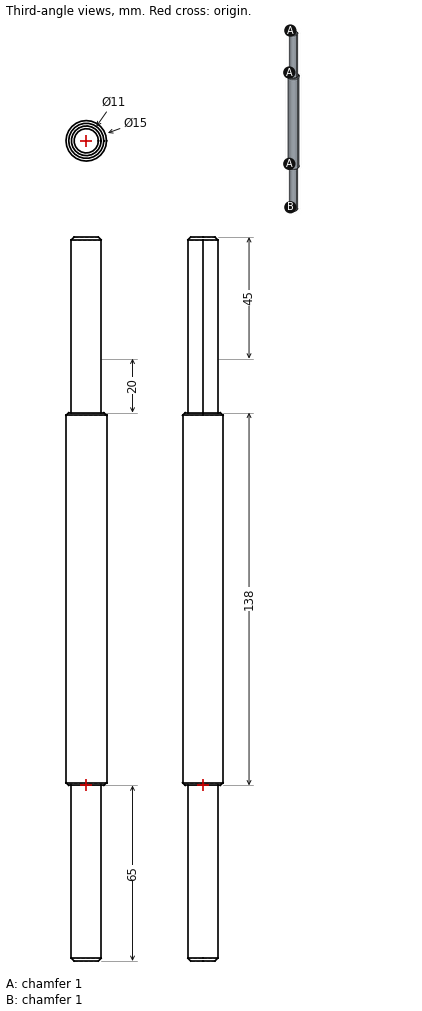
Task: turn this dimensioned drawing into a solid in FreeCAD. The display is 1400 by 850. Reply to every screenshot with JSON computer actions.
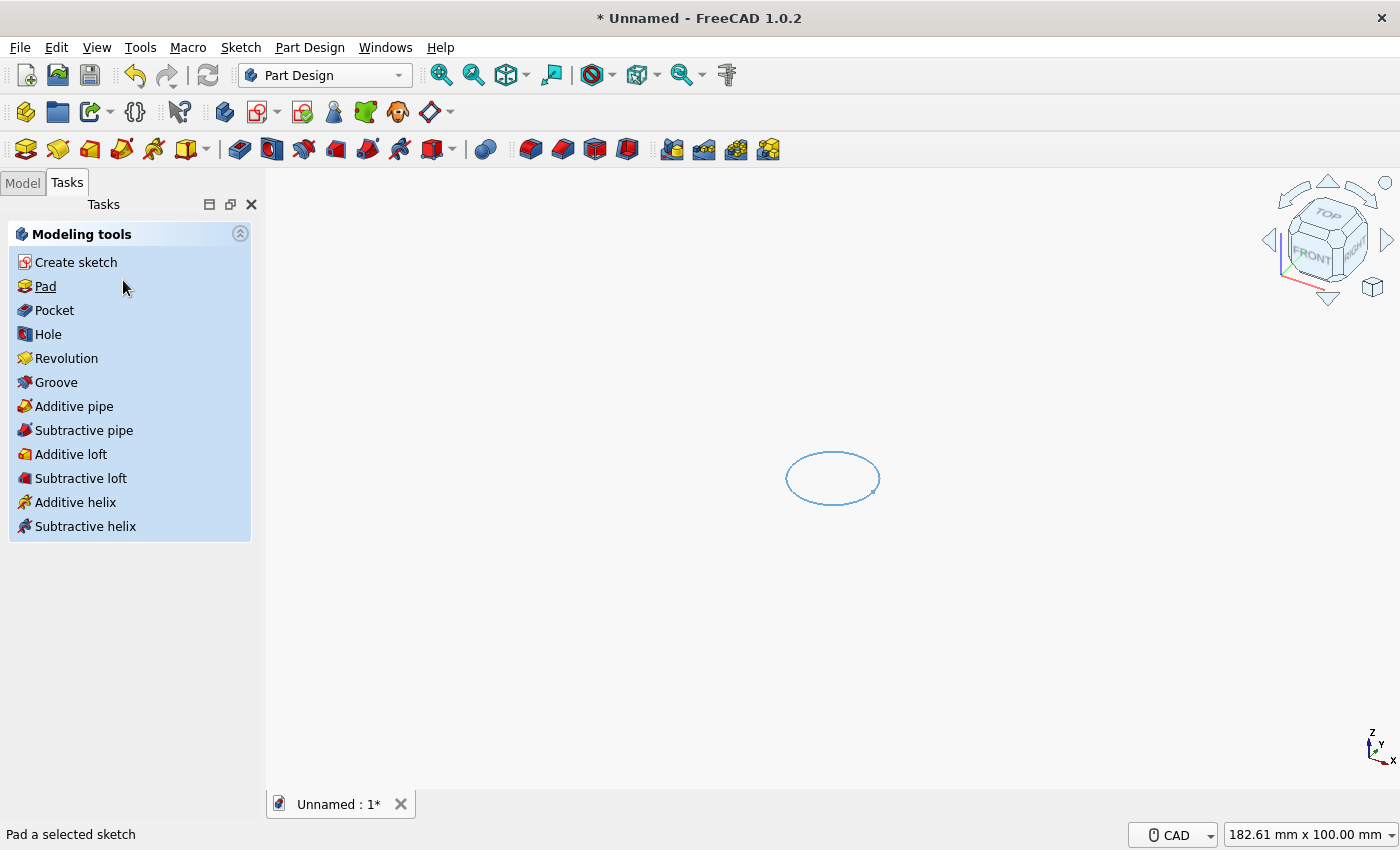
{"action": "left_click", "coordinate": [26, 150]}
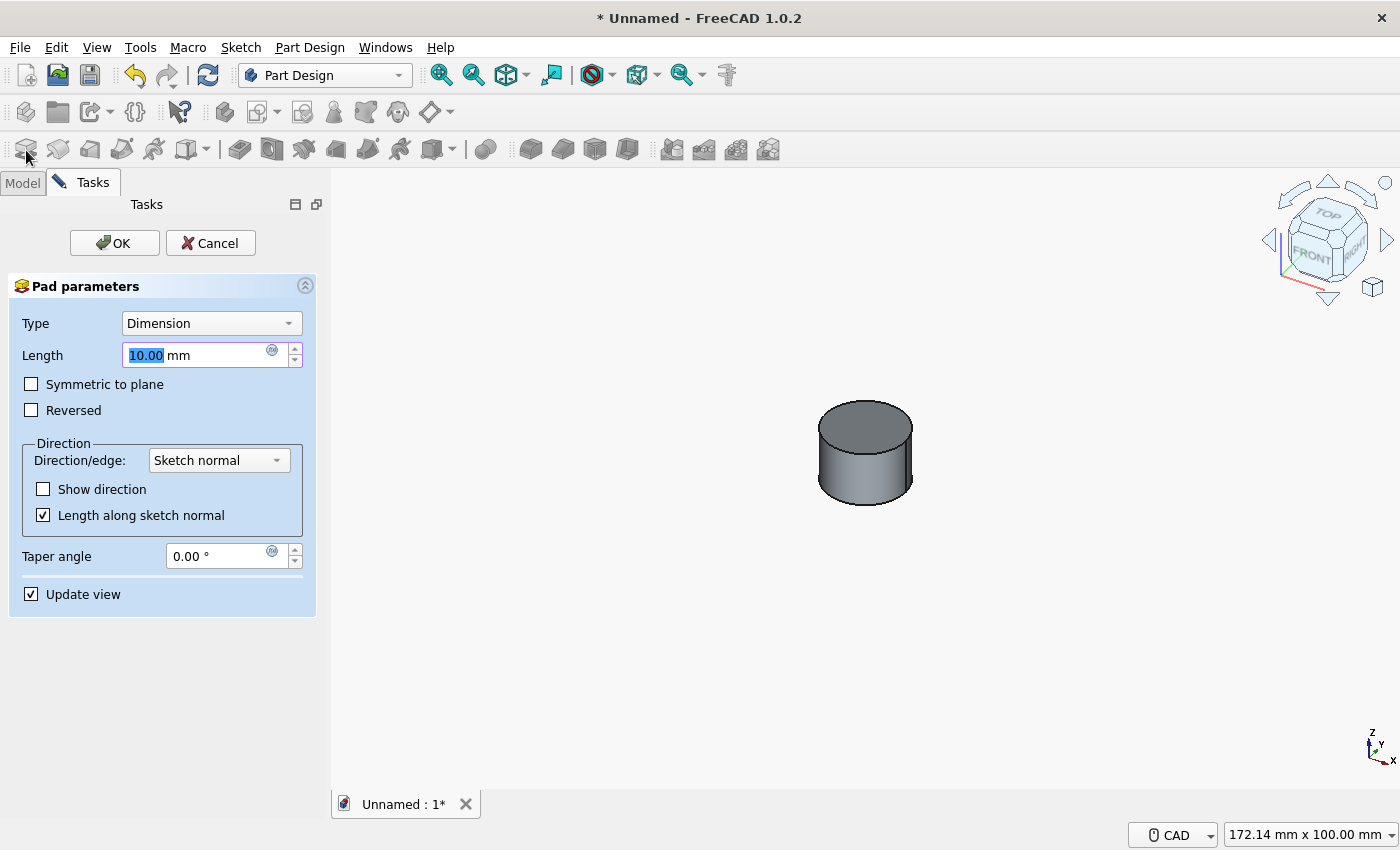
{"action": "type", "text": "138"}
{"action": "key", "text": "Tab"}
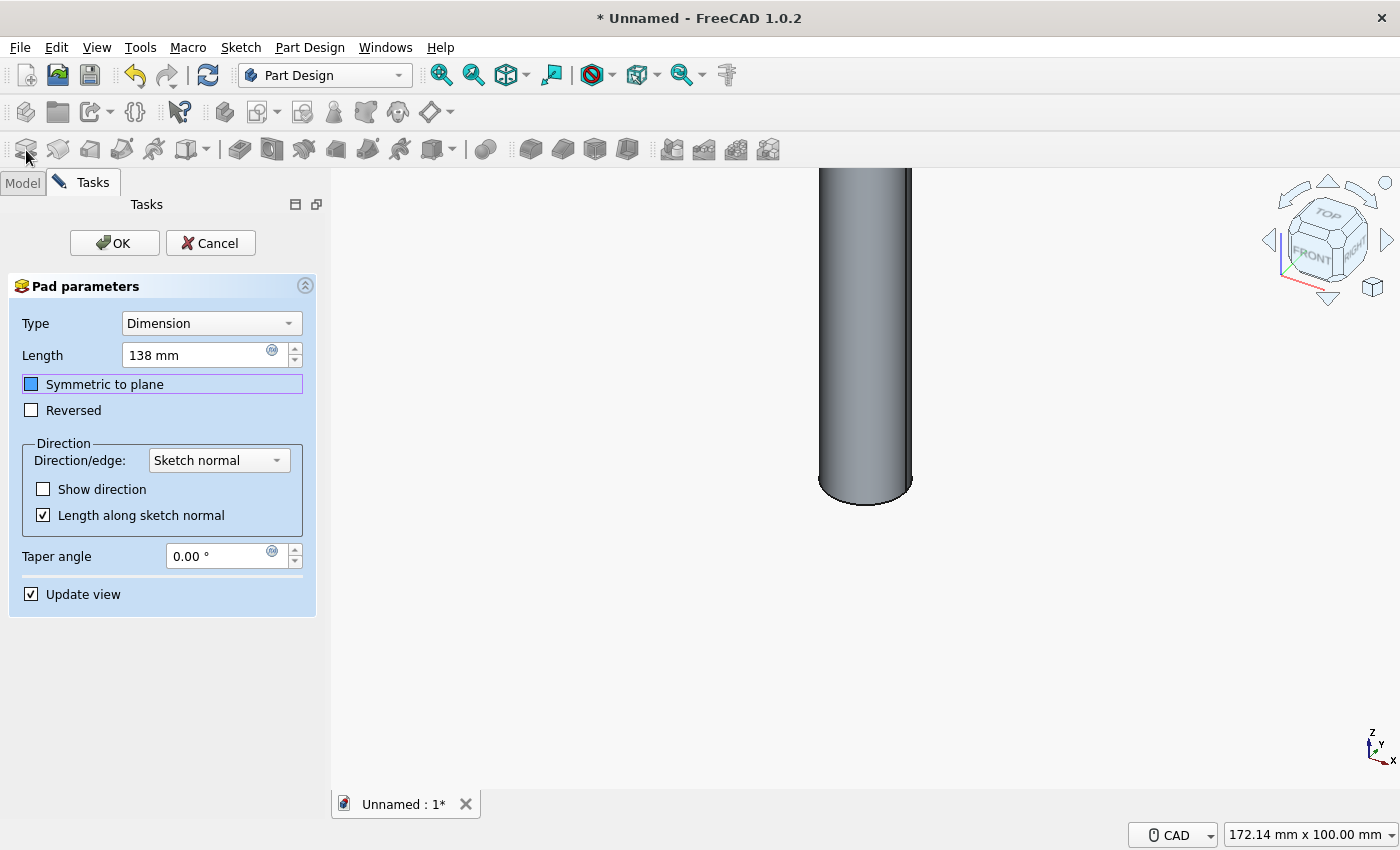
{"action": "left_click", "coordinate": [115, 243]}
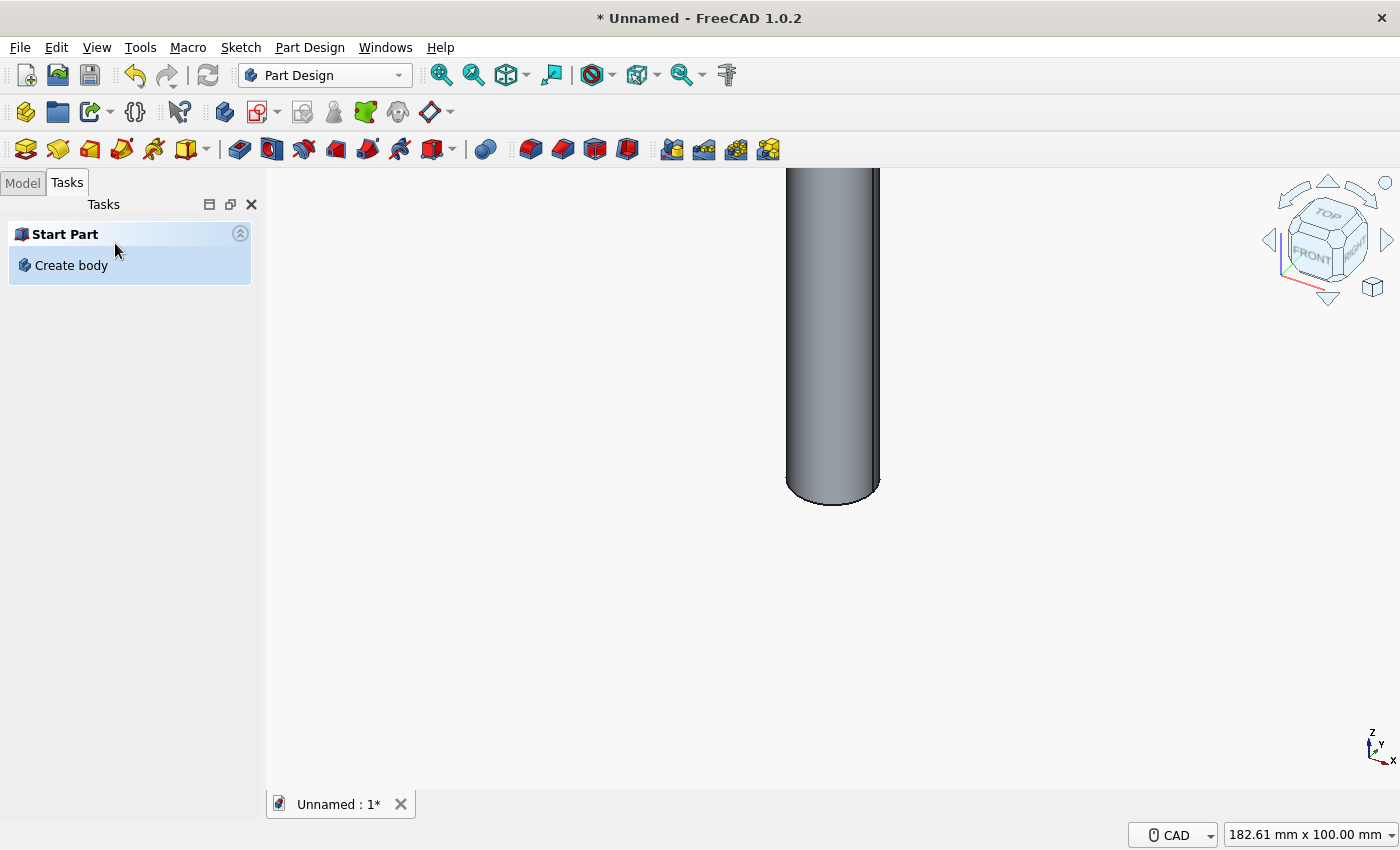
{"action": "key", "text": "v f"}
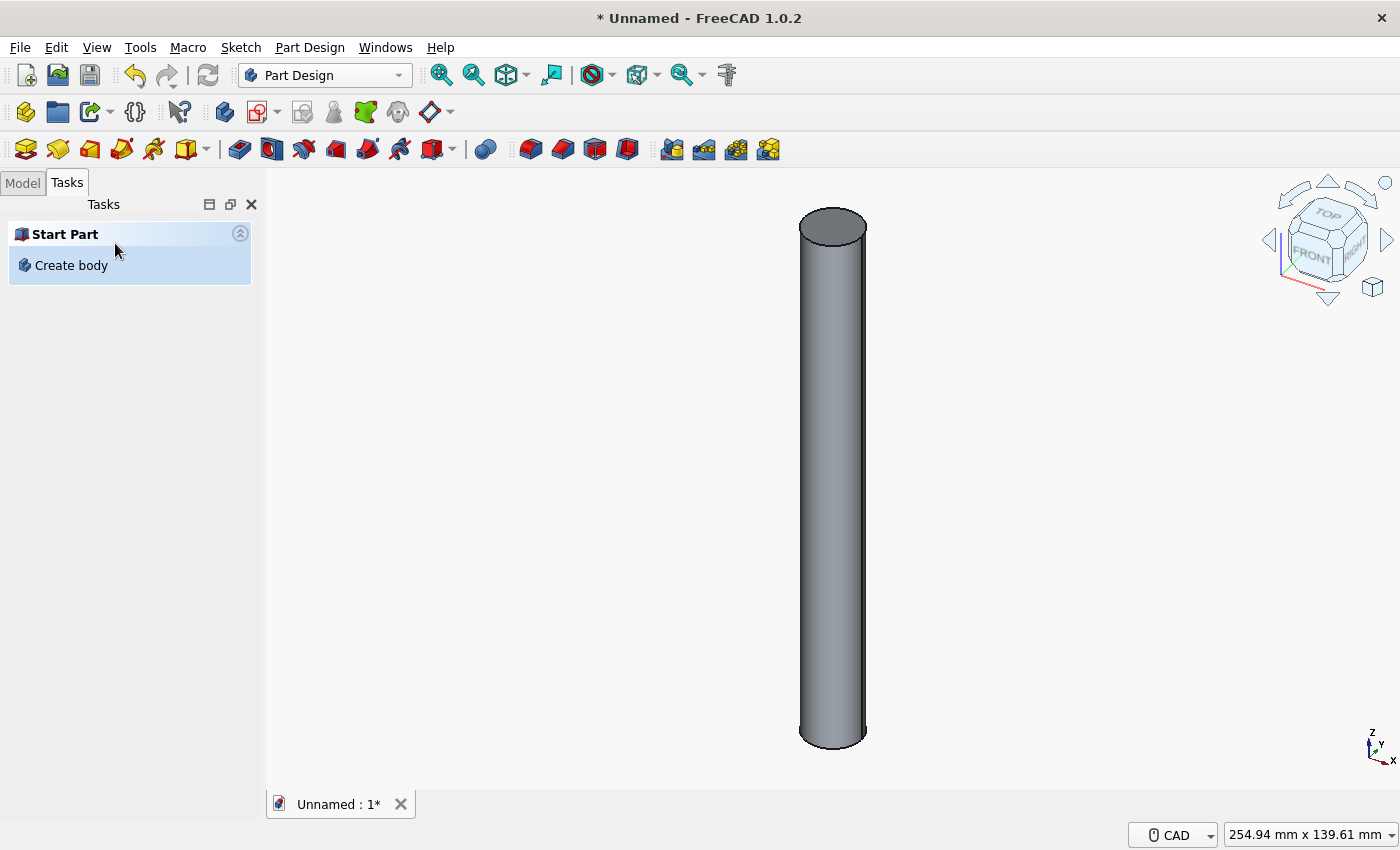
{"action": "left_click", "coordinate": [833, 226]}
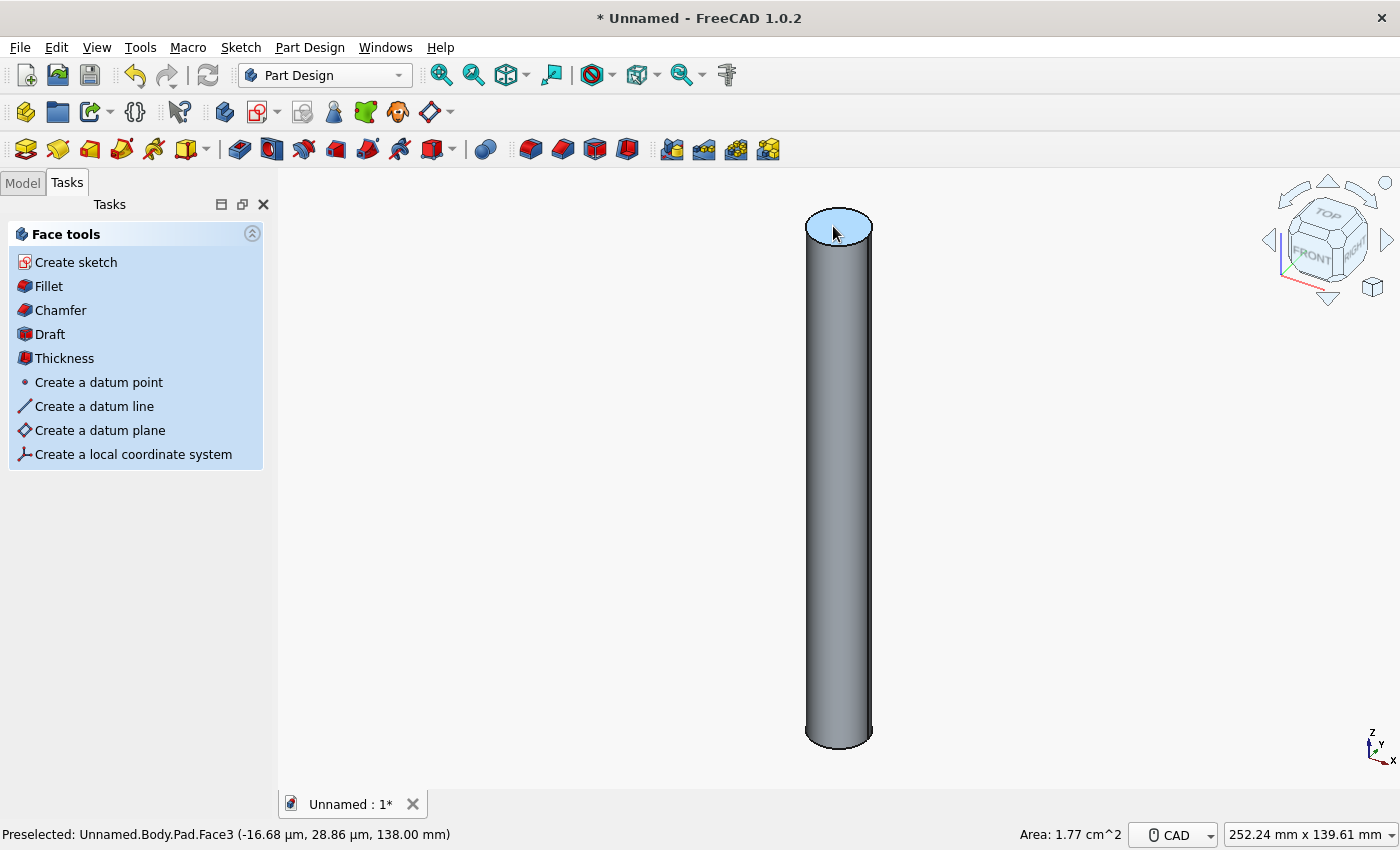
{"action": "left_click", "coordinate": [258, 112]}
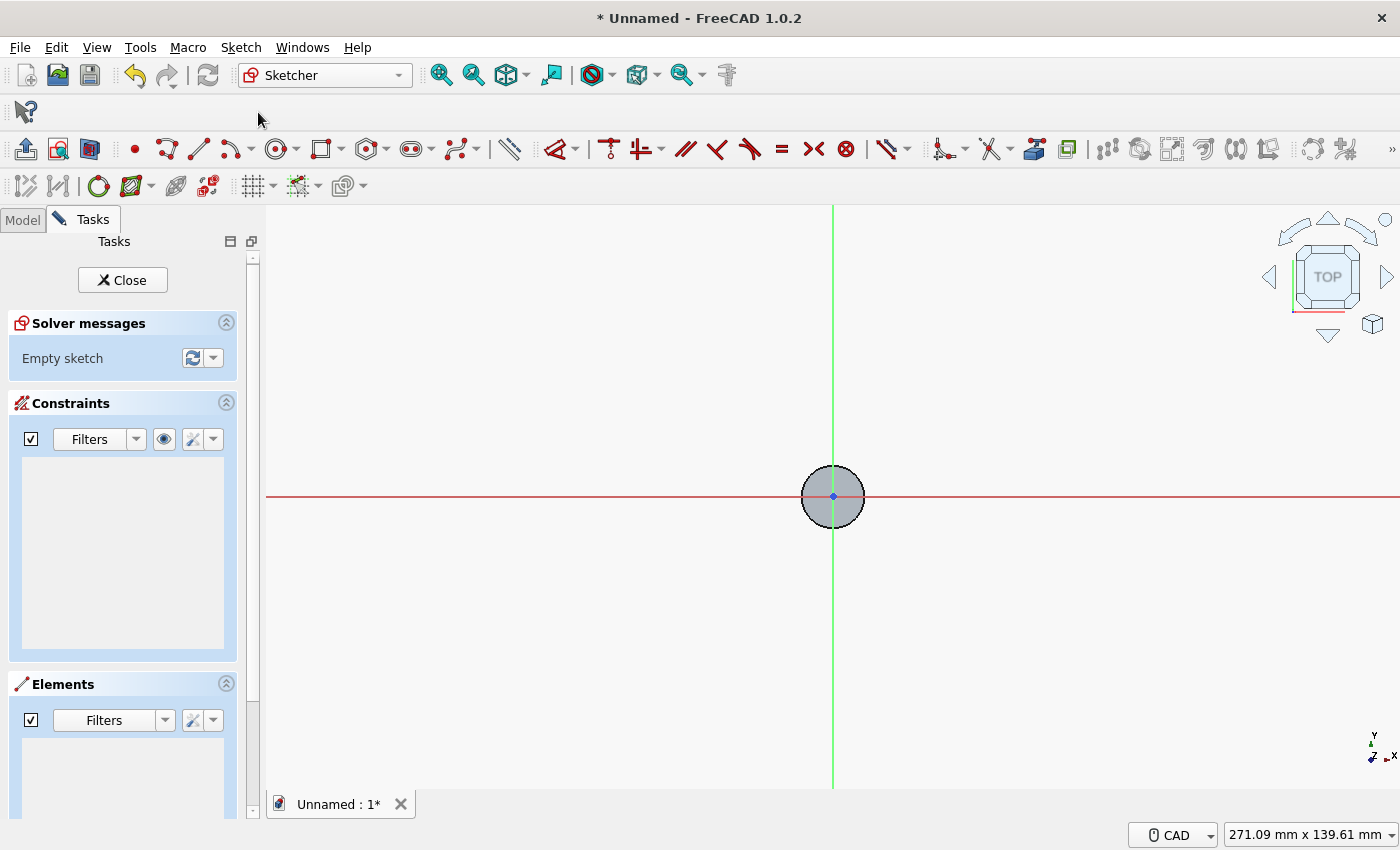
{"action": "scroll", "coordinate": [844, 497], "scroll_direction": "up", "scroll_amount": 10}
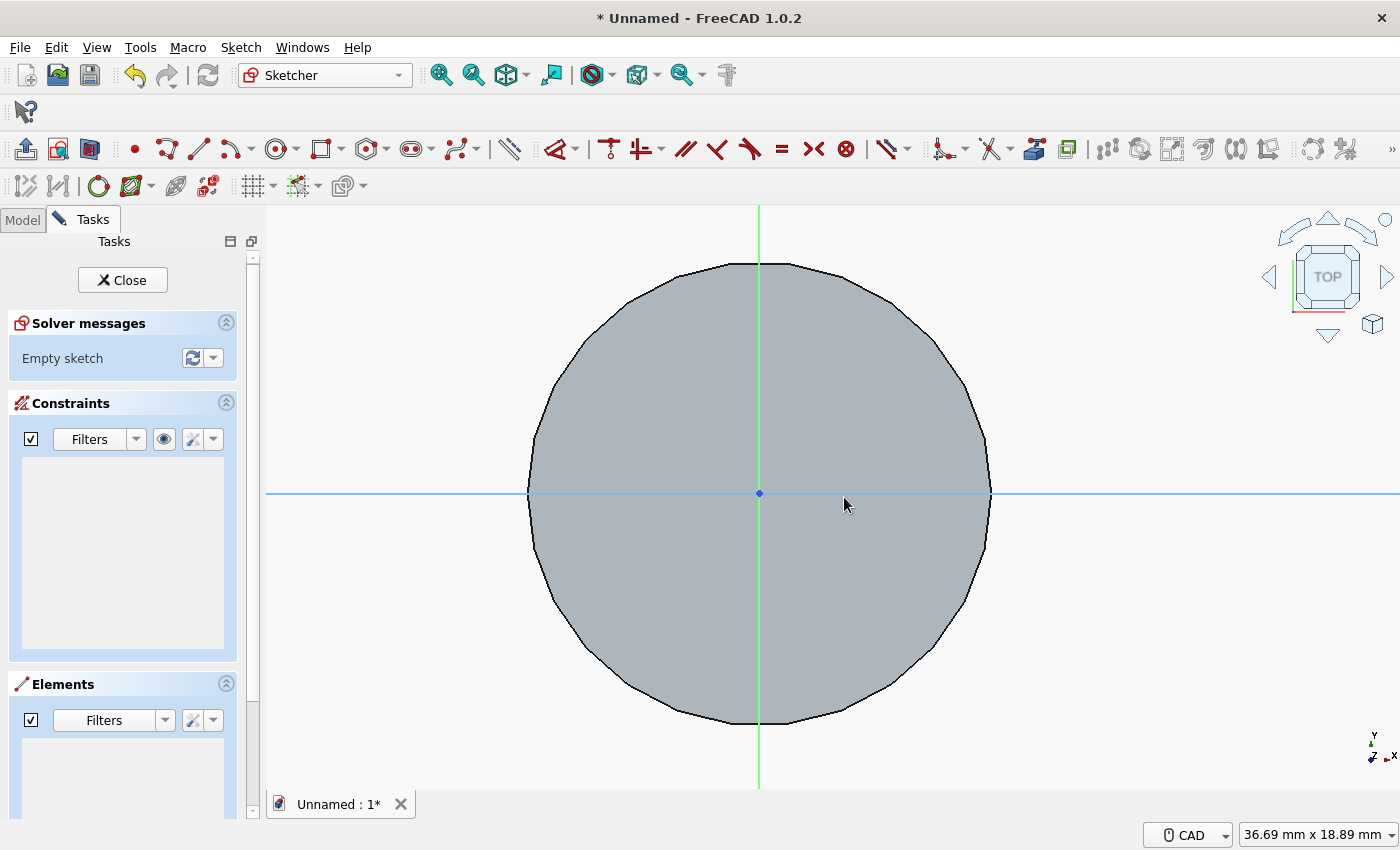
{"action": "key", "text": "g c"}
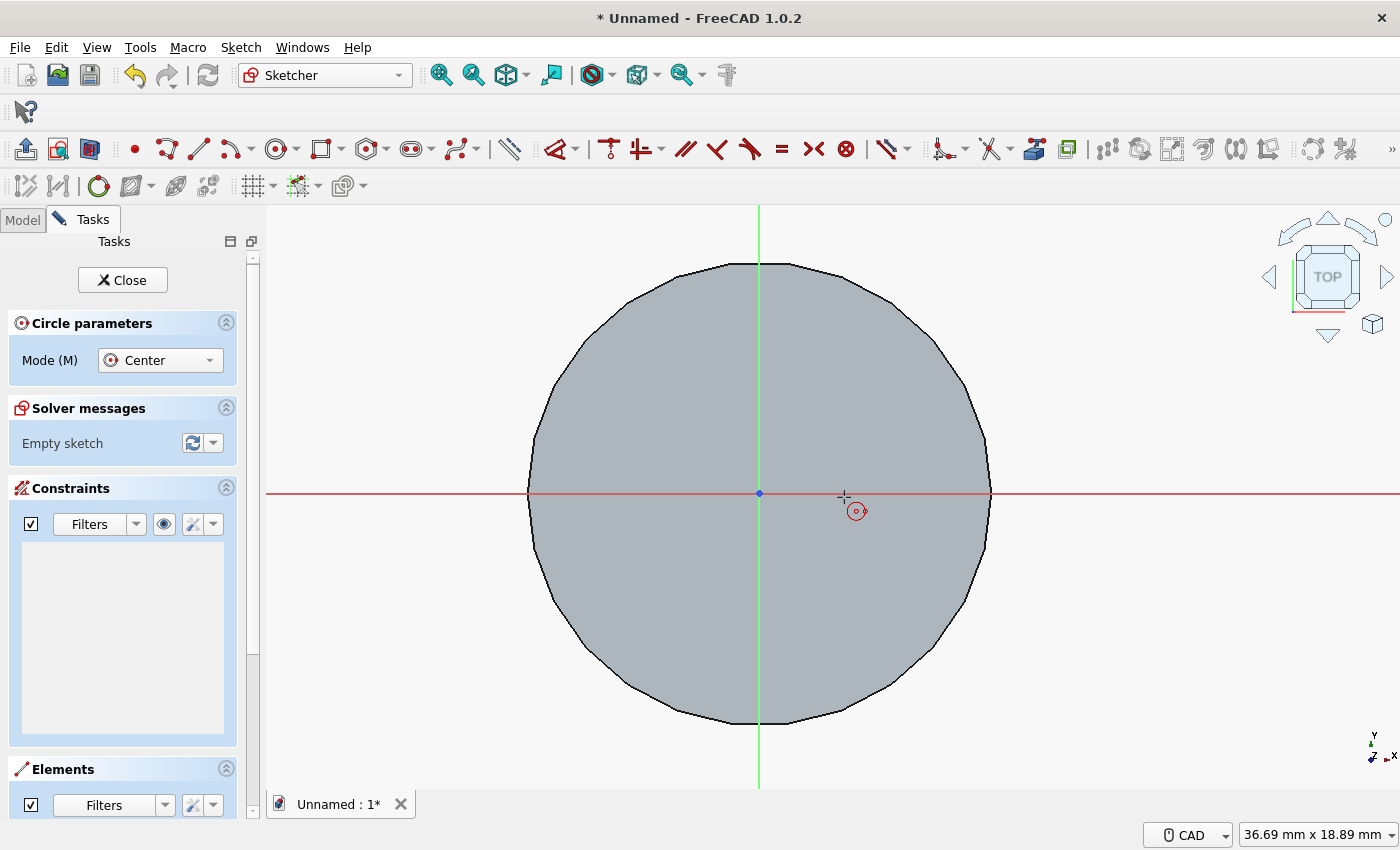
{"action": "left_click", "coordinate": [759, 494]}
{"action": "mouse_move", "coordinate": [880, 374]}